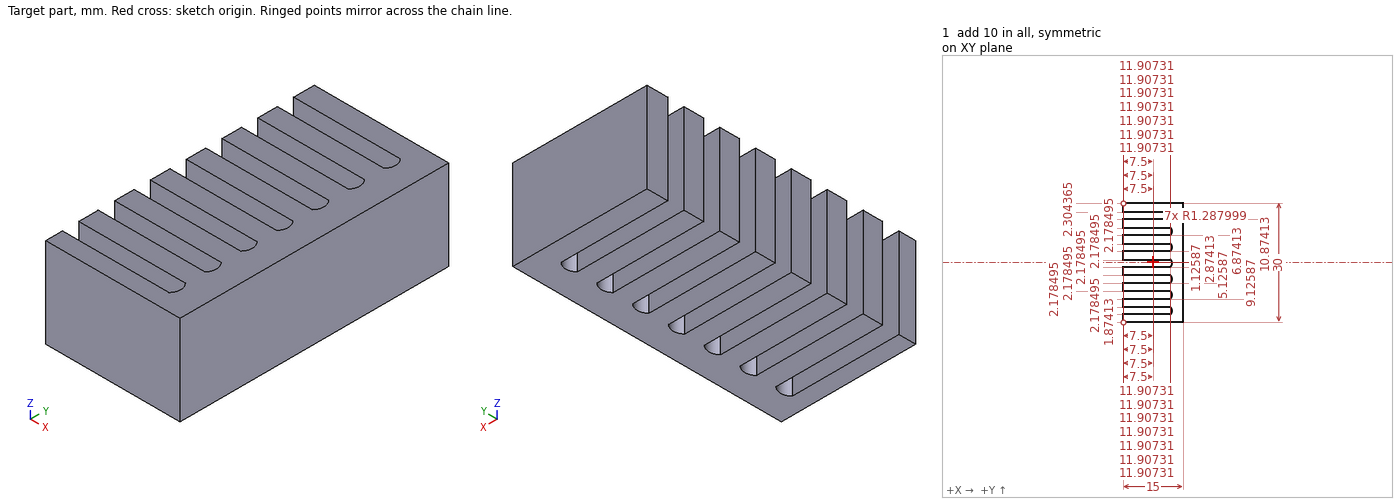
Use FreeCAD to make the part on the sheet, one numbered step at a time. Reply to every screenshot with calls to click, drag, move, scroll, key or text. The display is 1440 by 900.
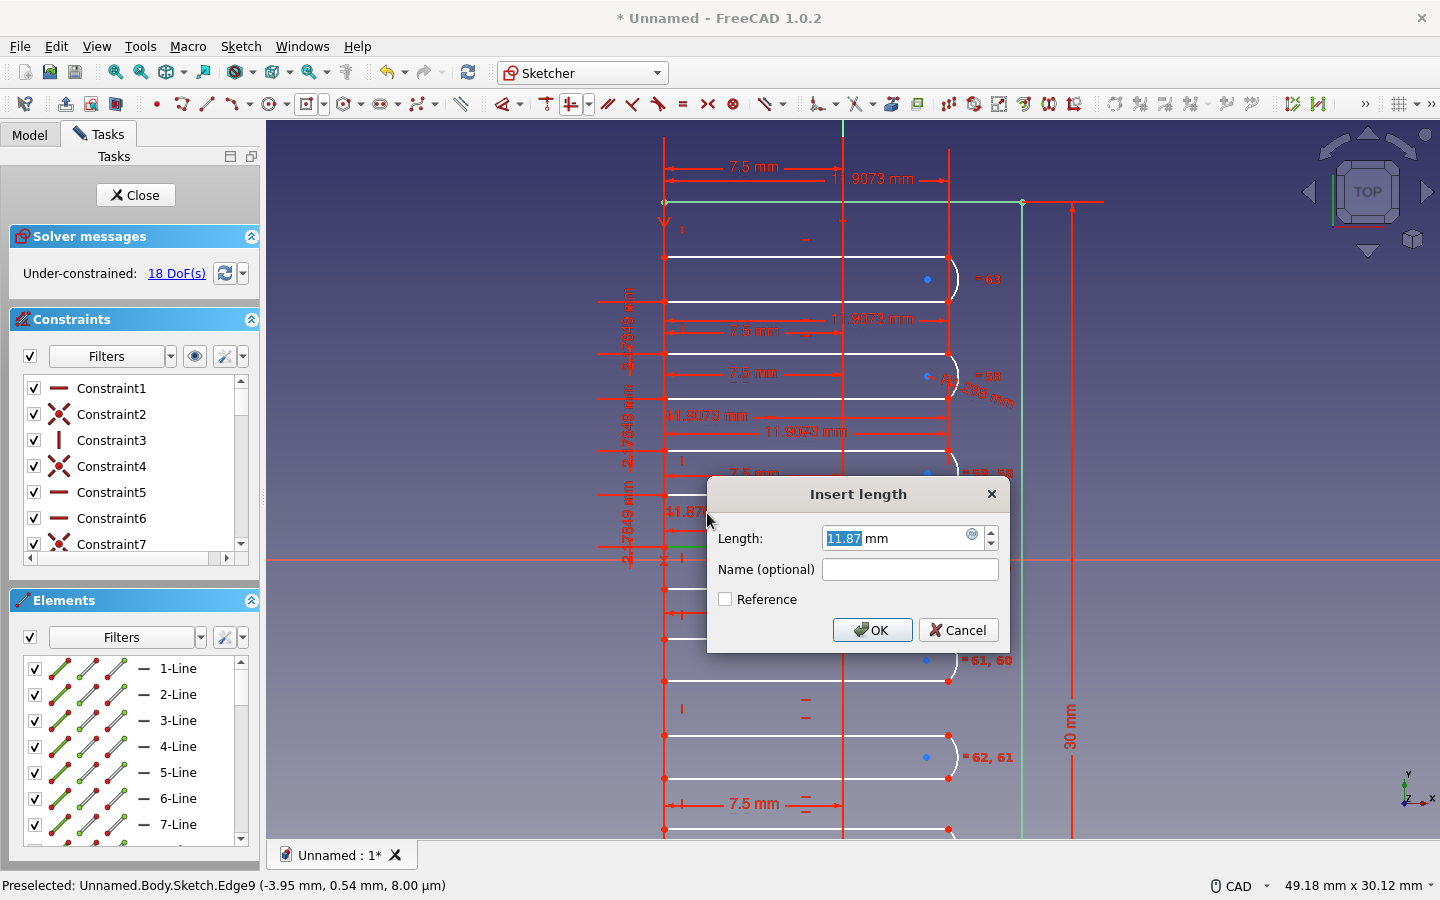
text(11.90731)
key(Return)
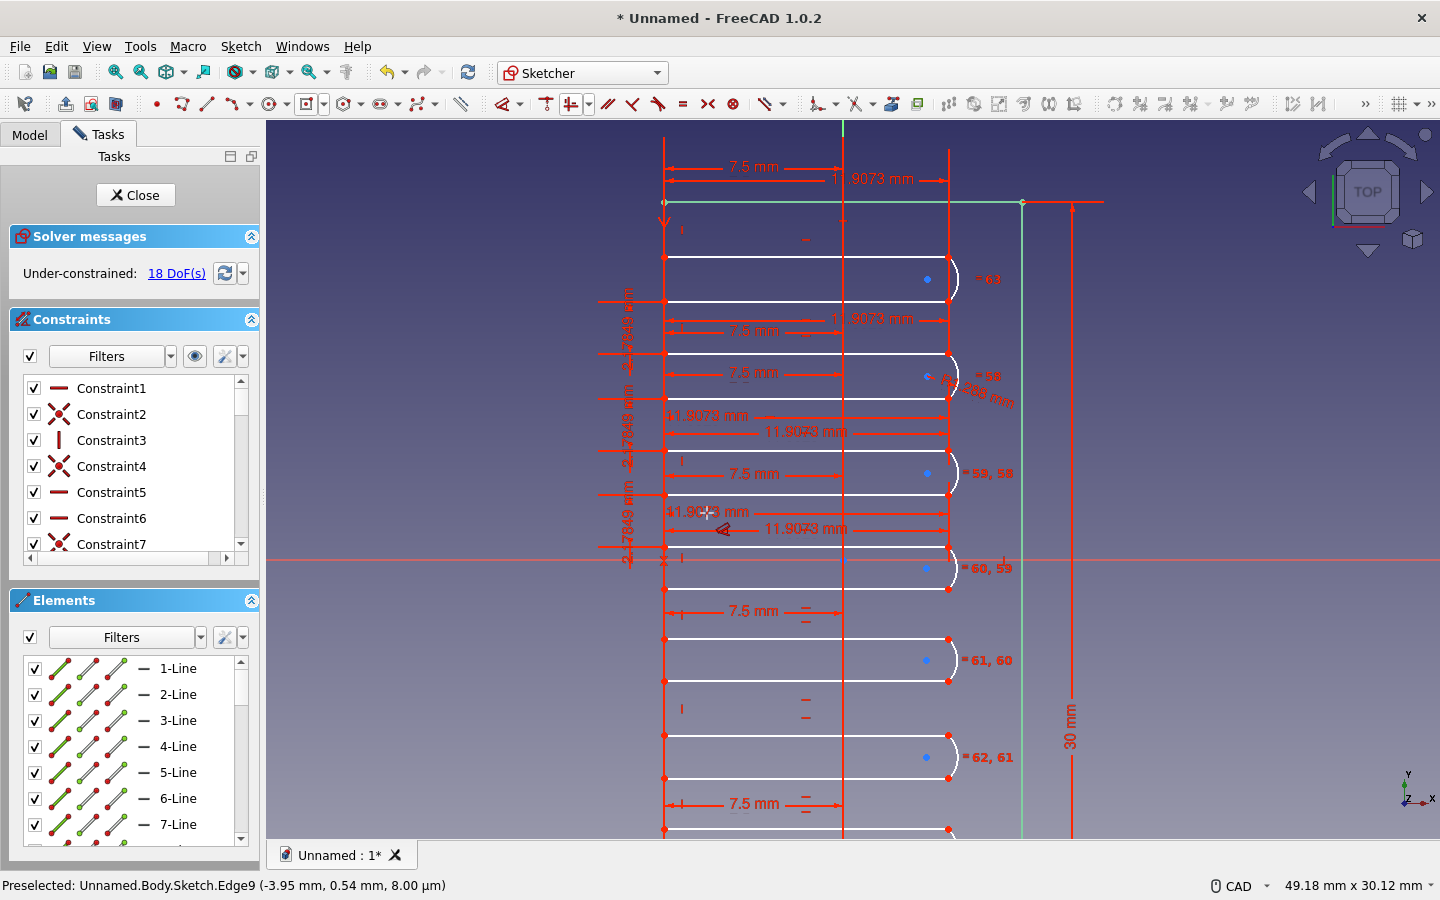
click(863, 589)
click(872, 623)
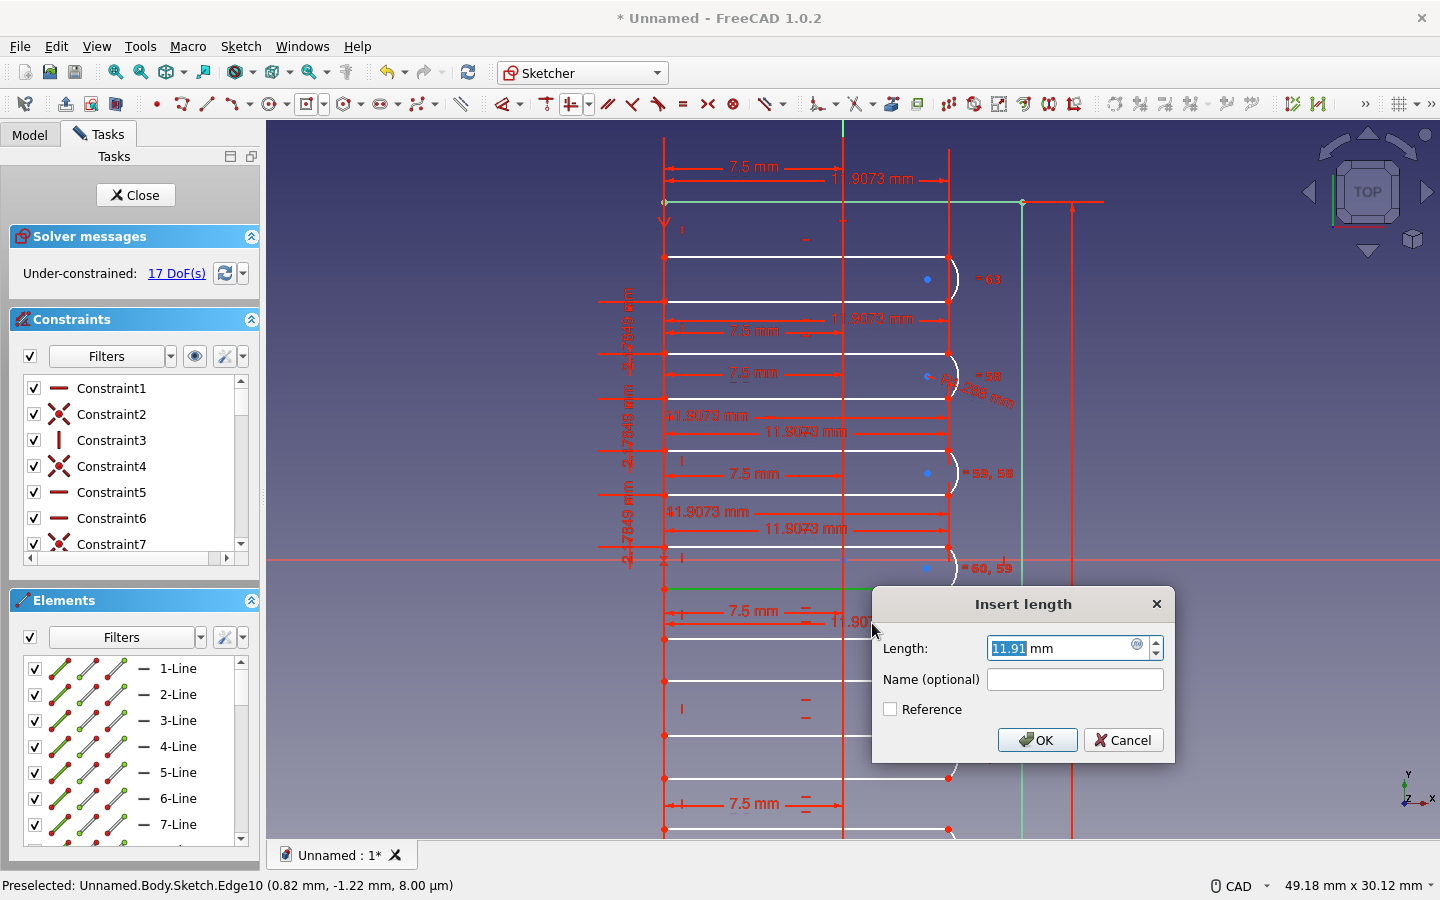
text(11.90731)
key(Return)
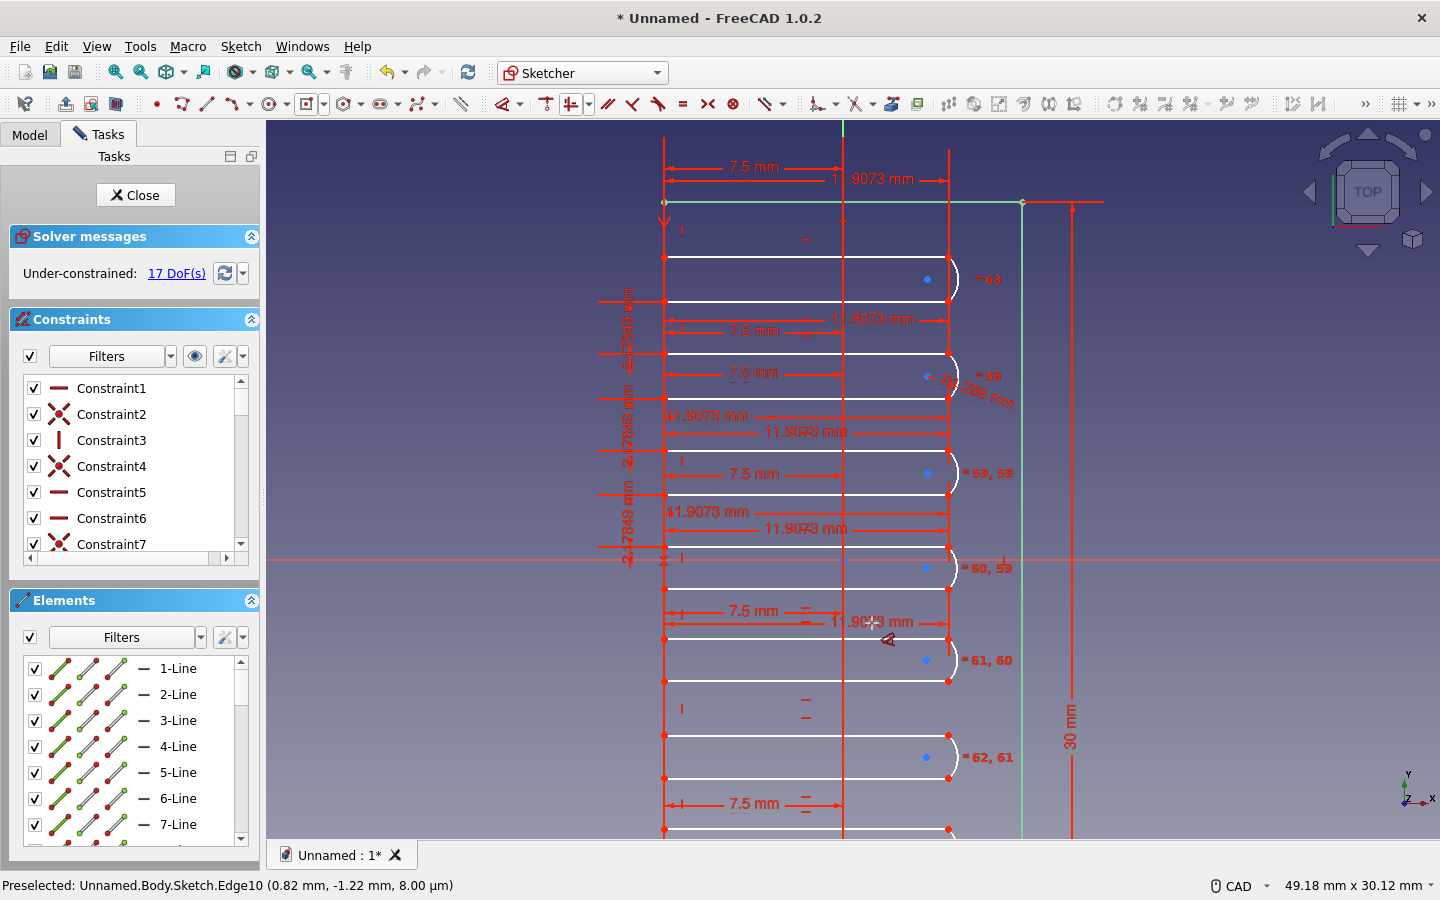
click(664, 604)
click(630, 614)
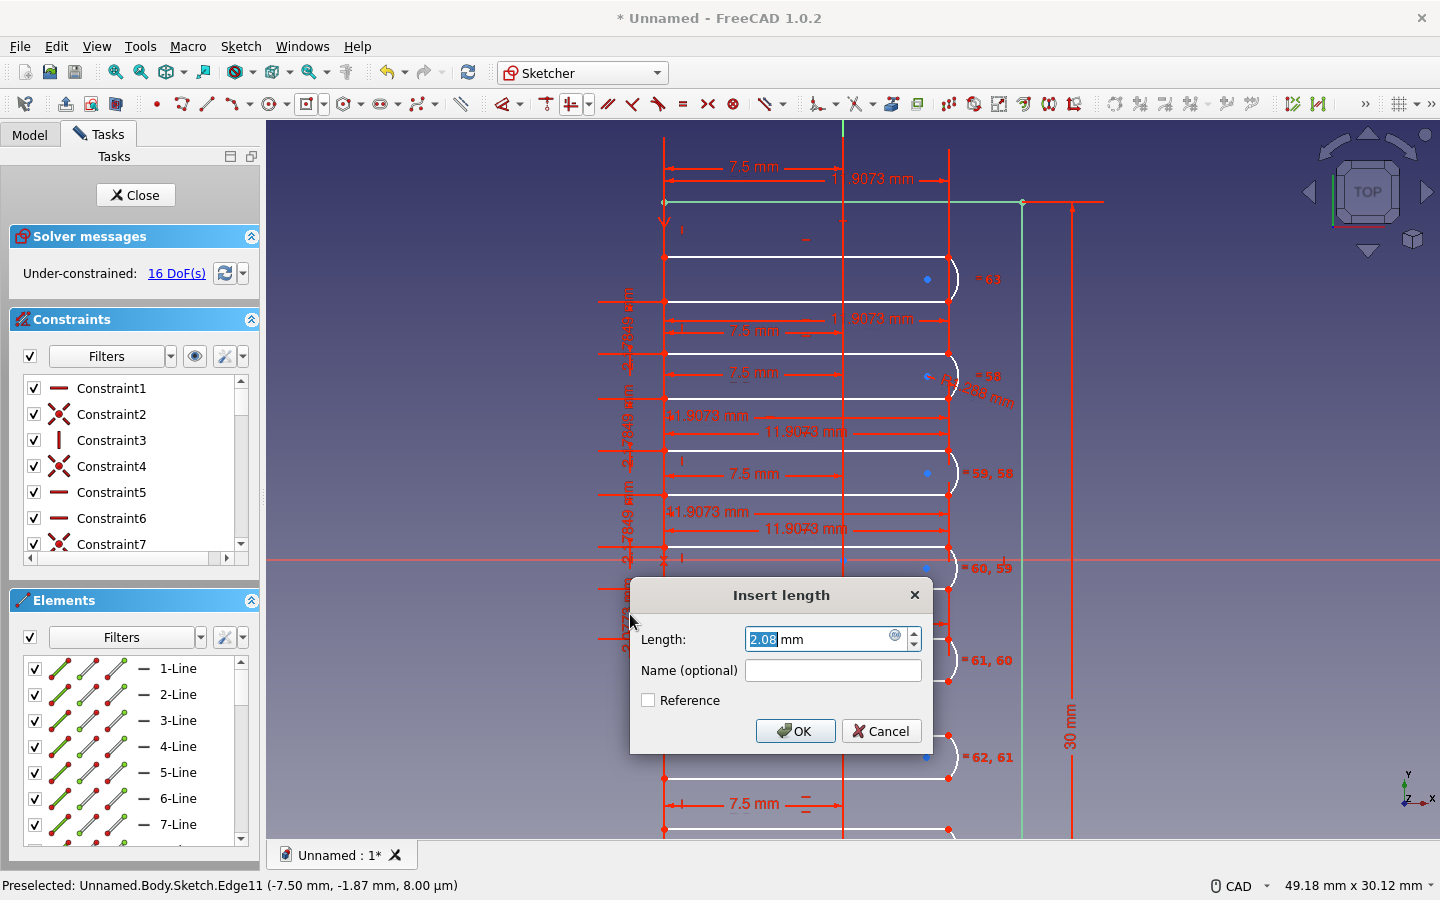
text(2.178495)
key(Return)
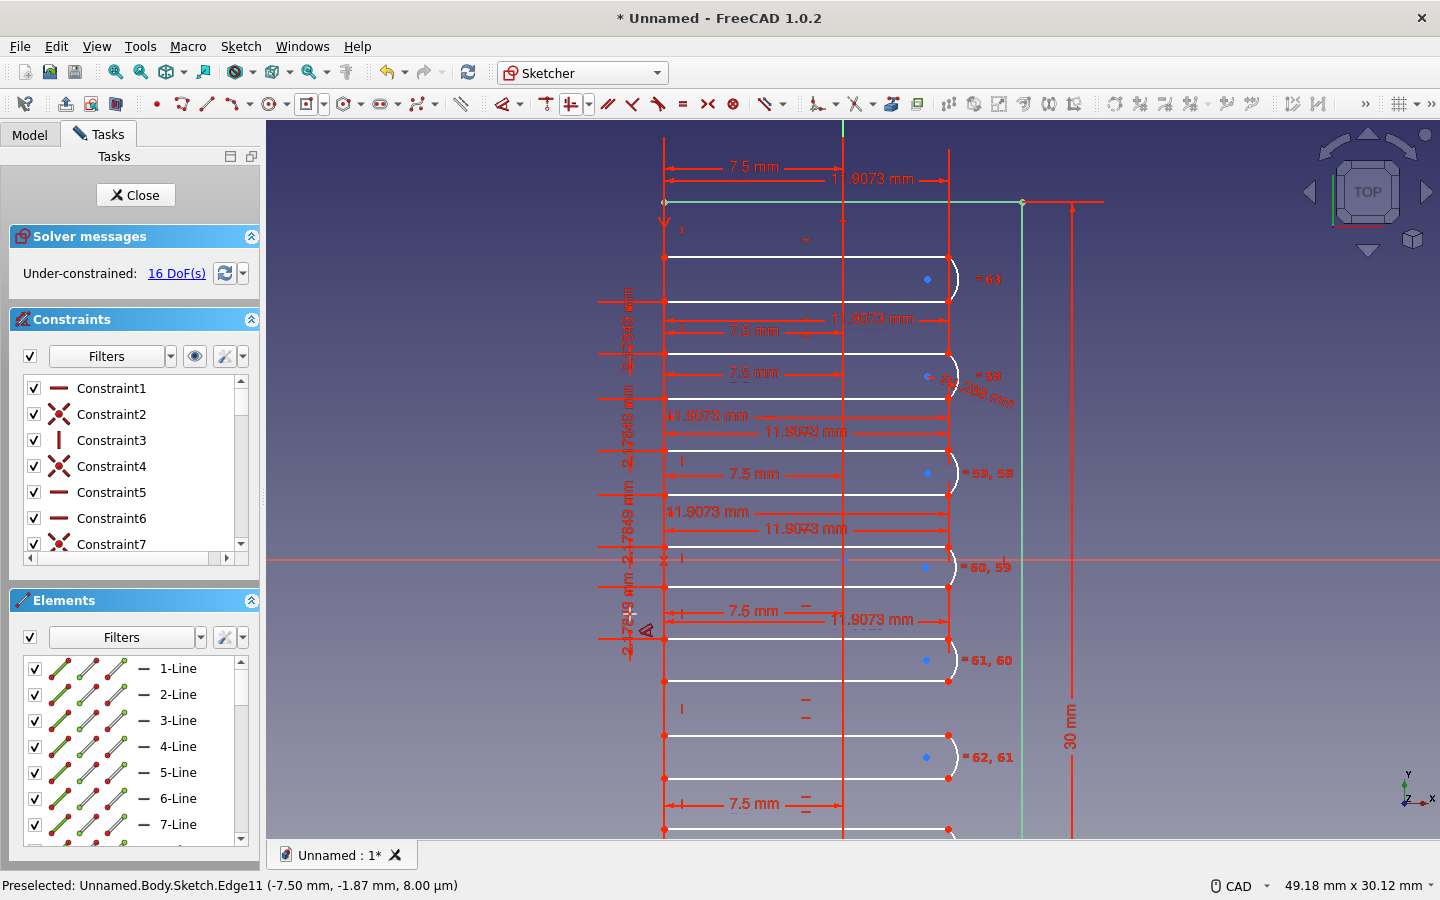
click(750, 639)
click(807, 697)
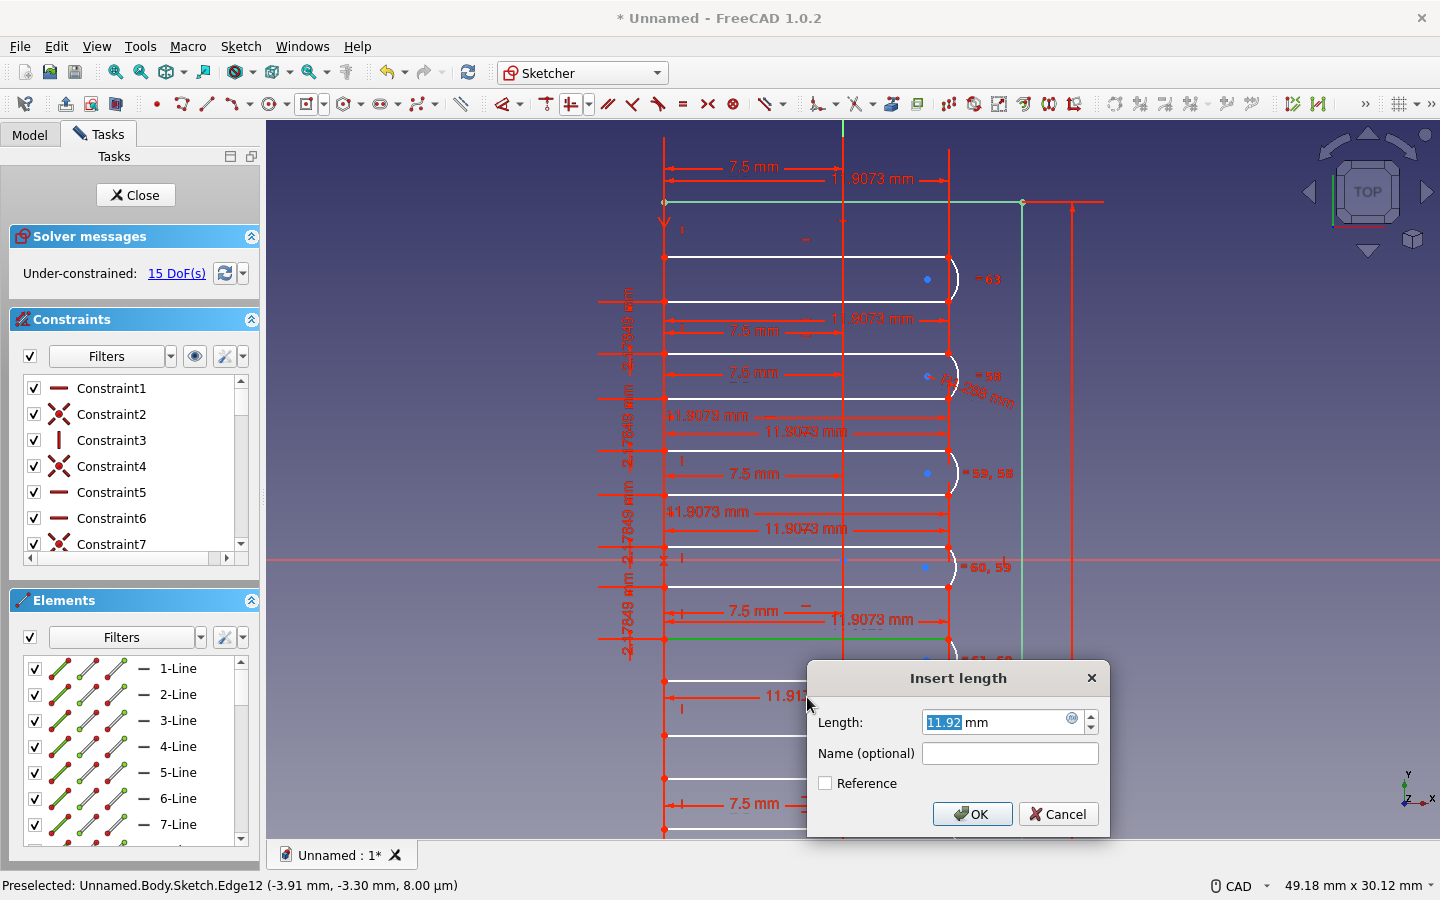
text(11.90731)
key(Return)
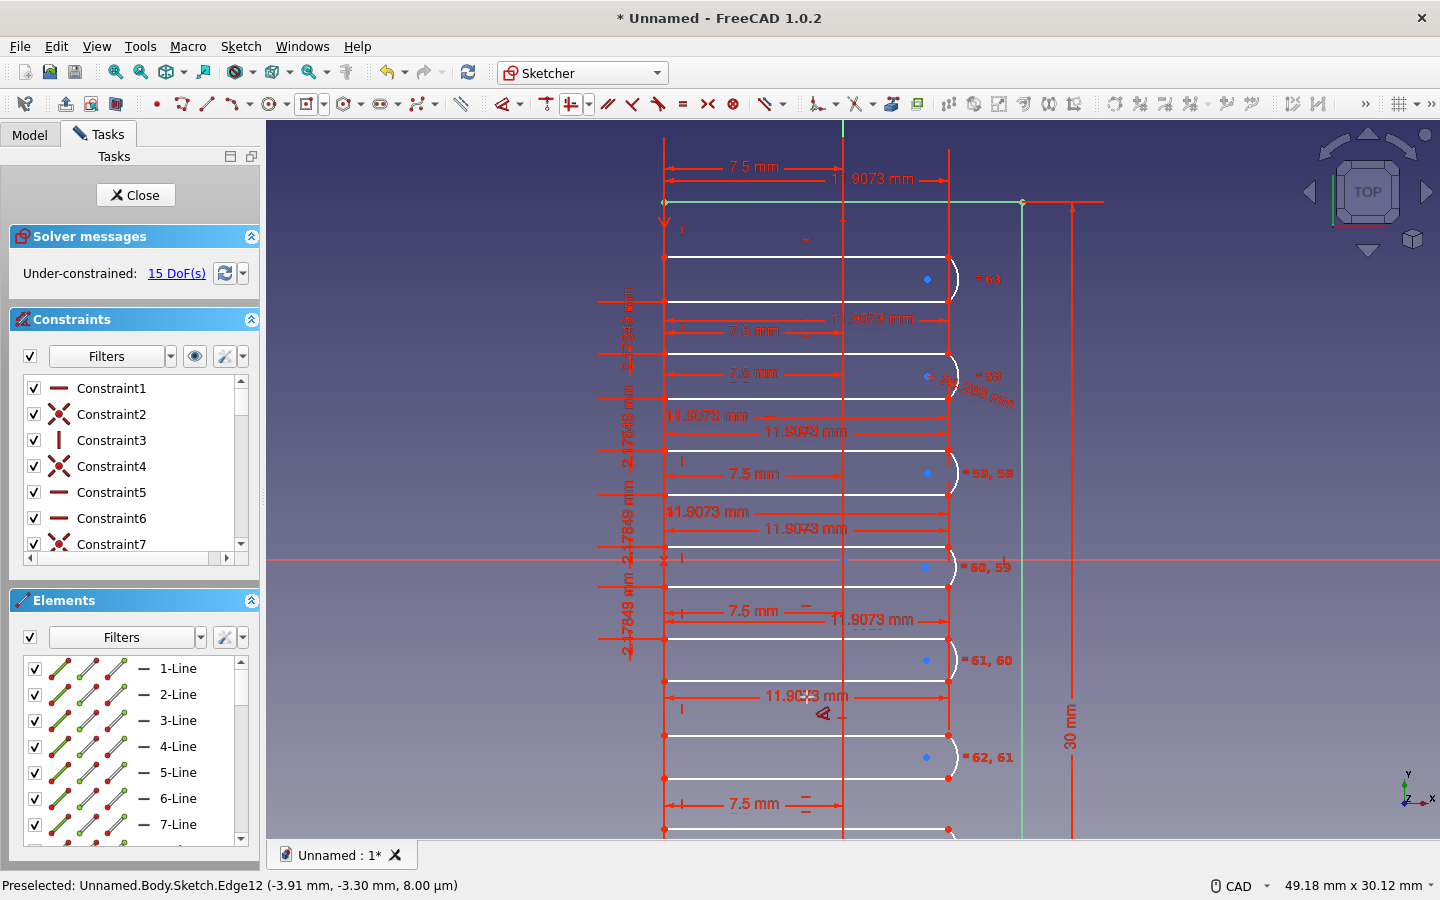
click(863, 681)
click(707, 715)